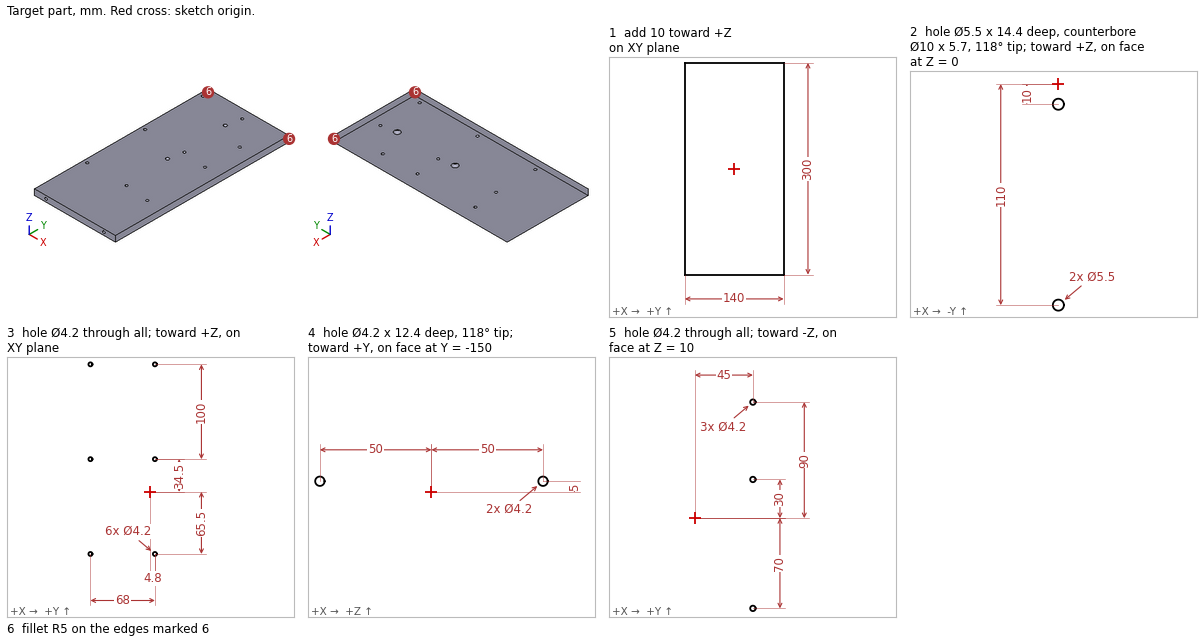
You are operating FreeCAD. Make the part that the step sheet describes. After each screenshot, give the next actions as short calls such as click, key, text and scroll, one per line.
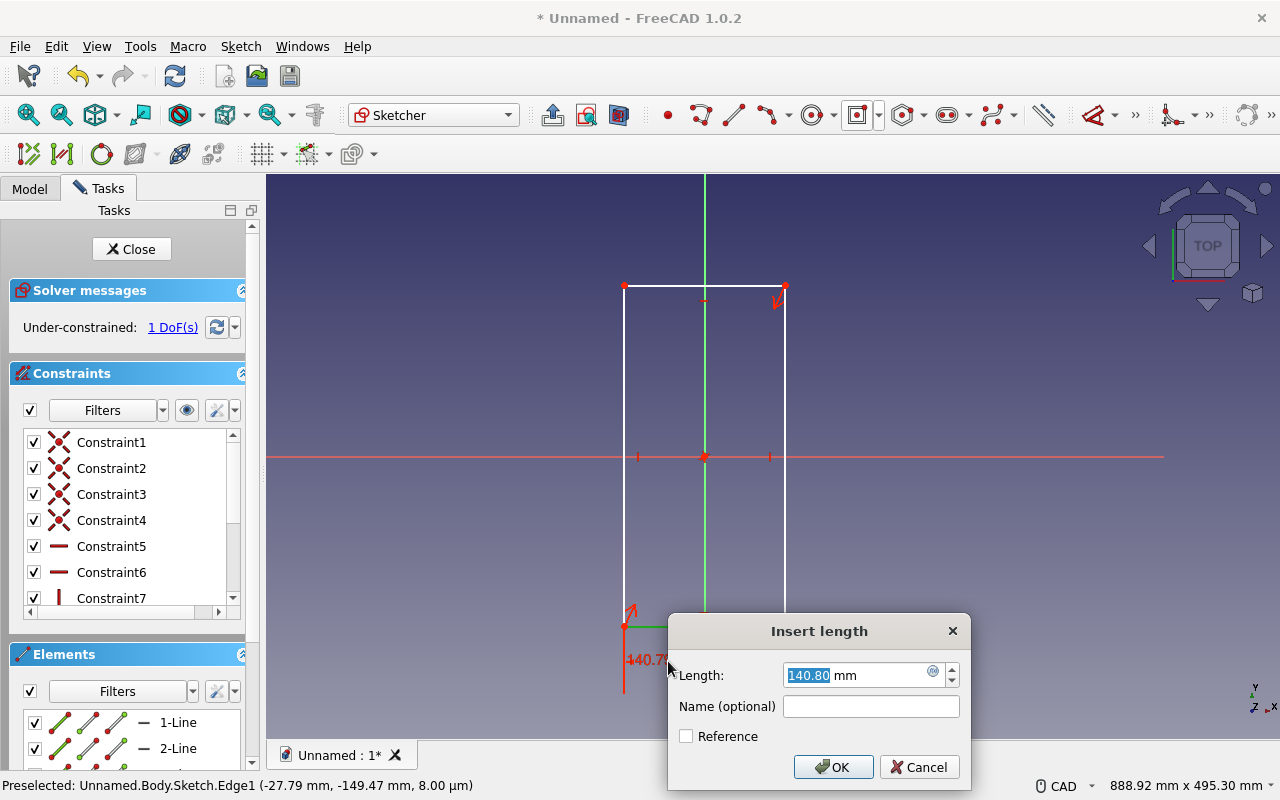
text(140)
key(Return)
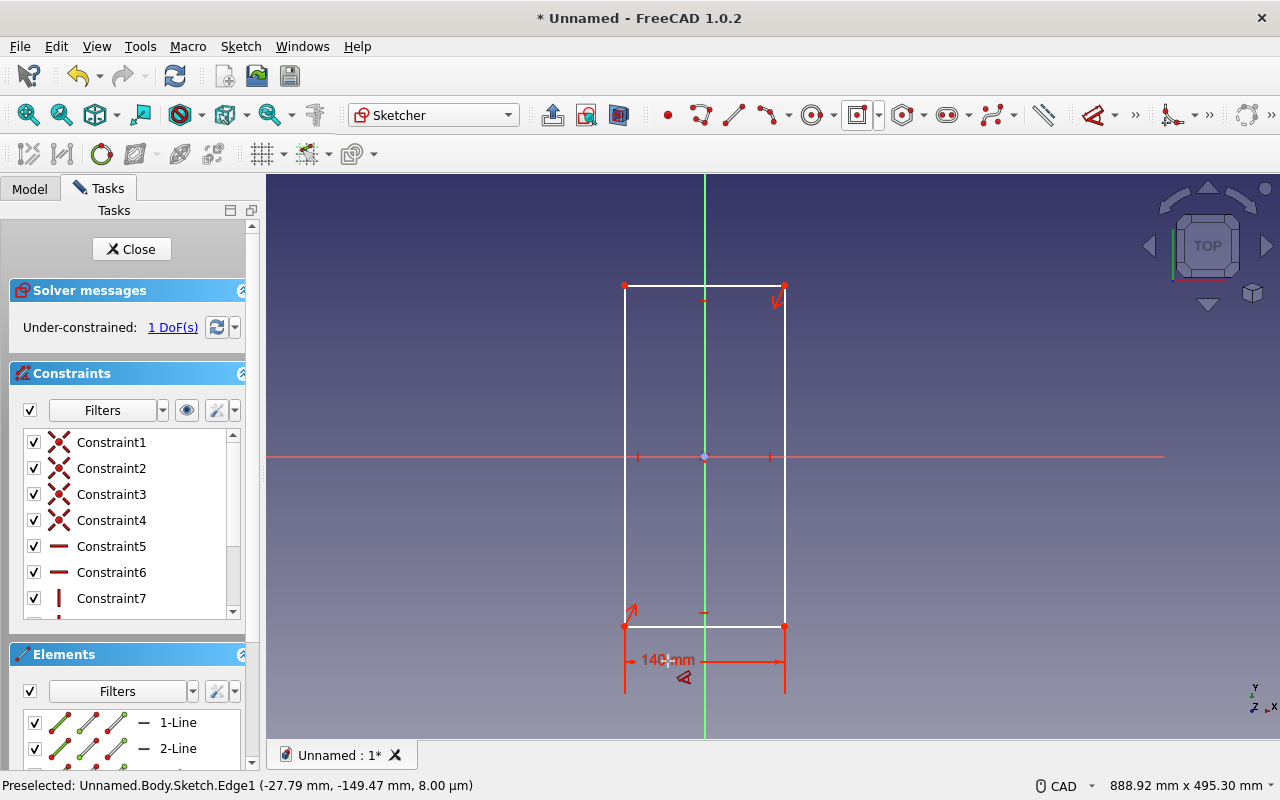
click(785, 525)
click(819, 378)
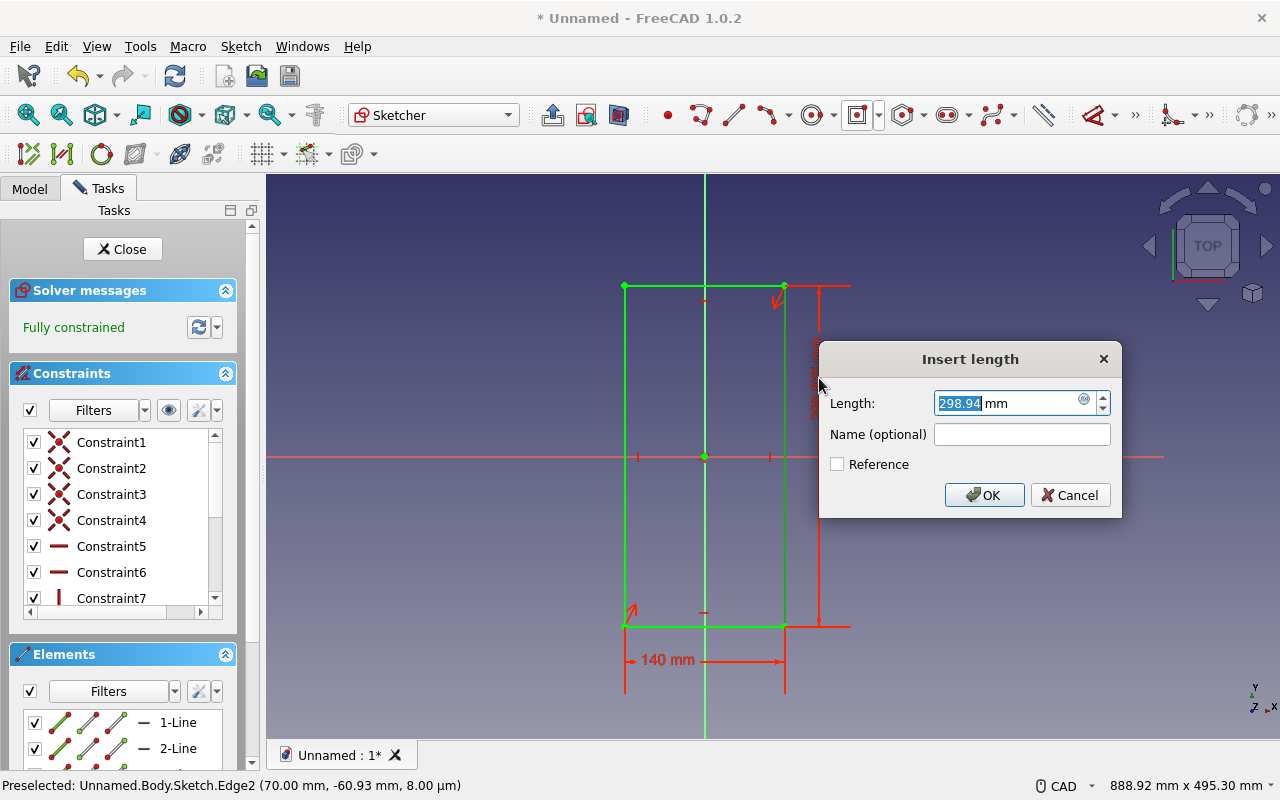
text(300)
key(Return)
key(Escape)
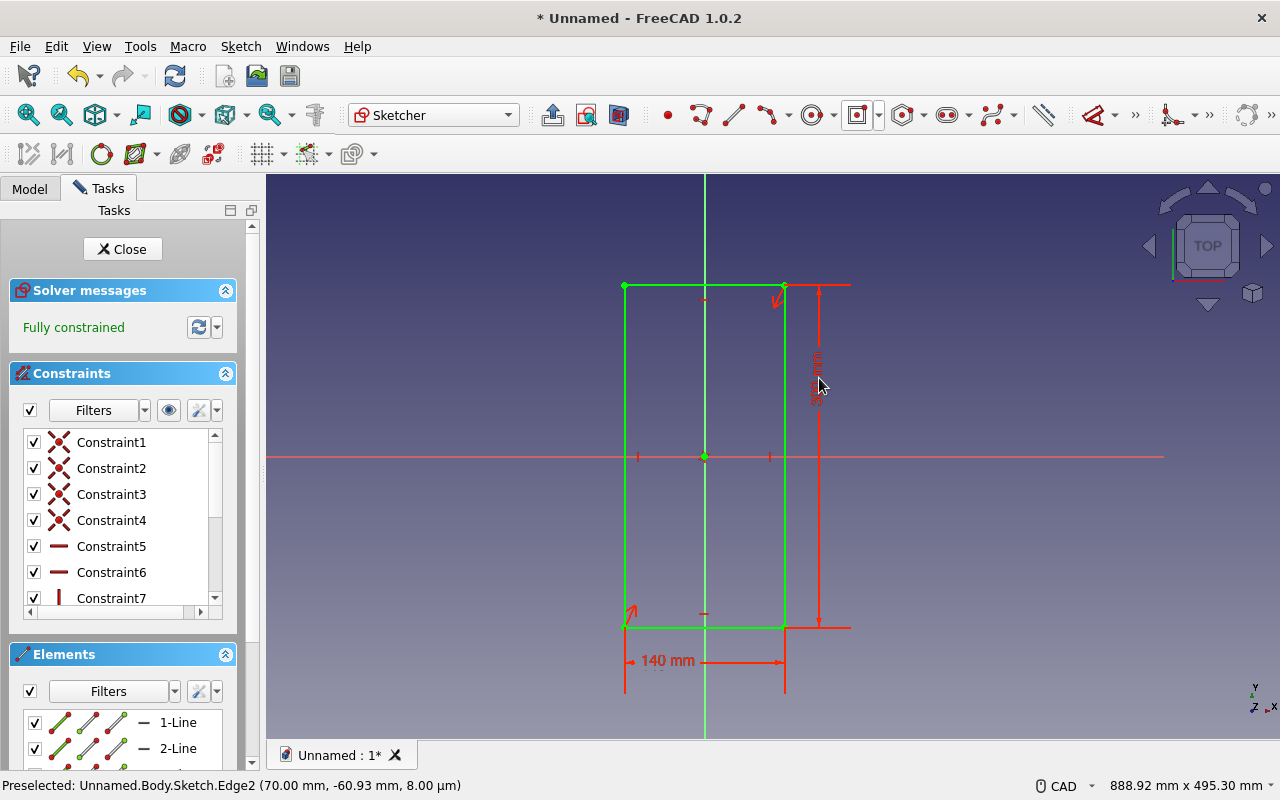
click(123, 249)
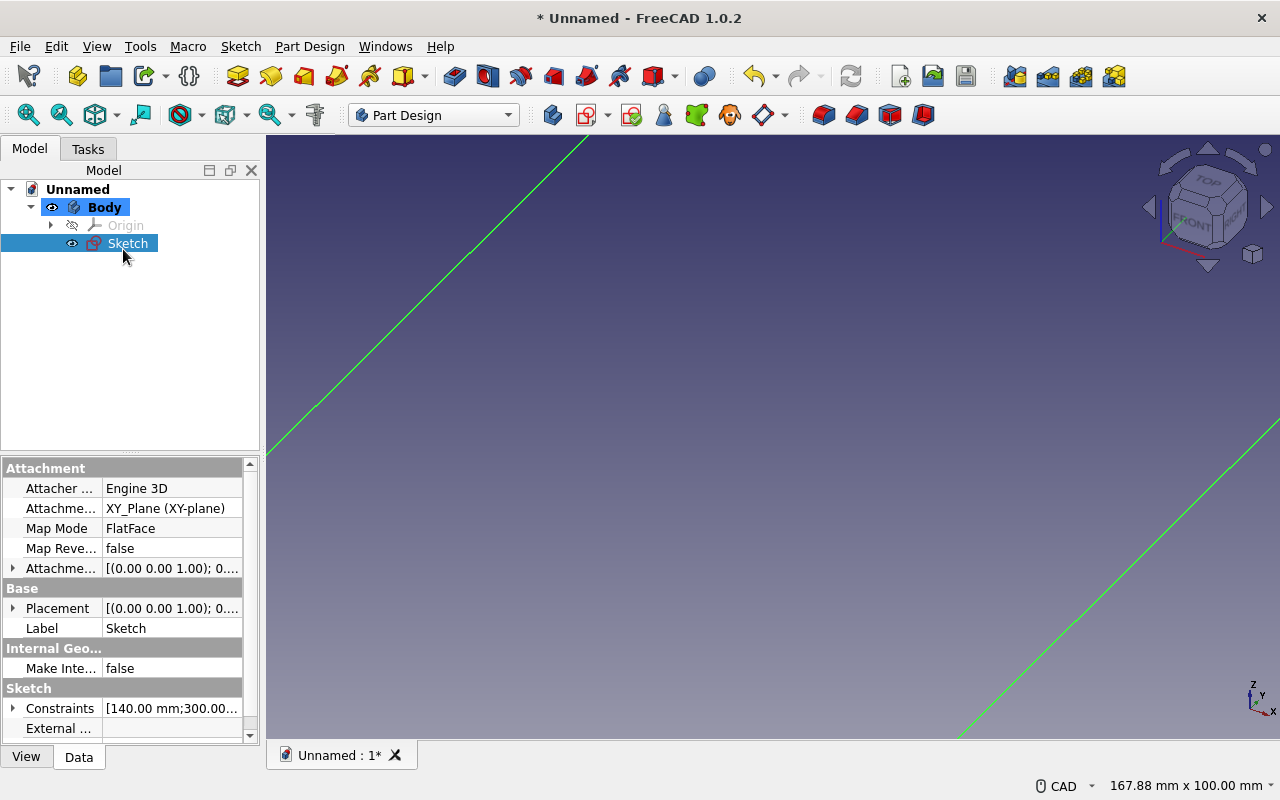
click(238, 76)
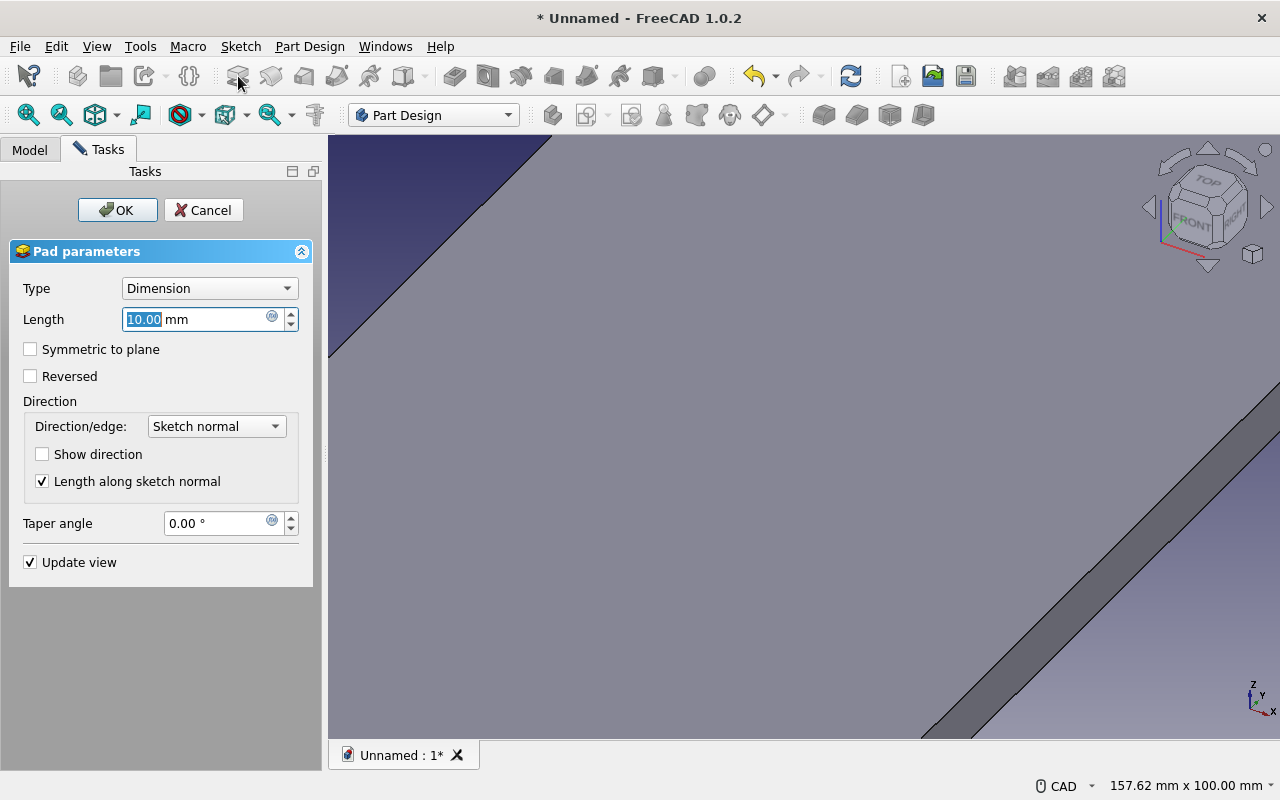
text(10)
key(Tab)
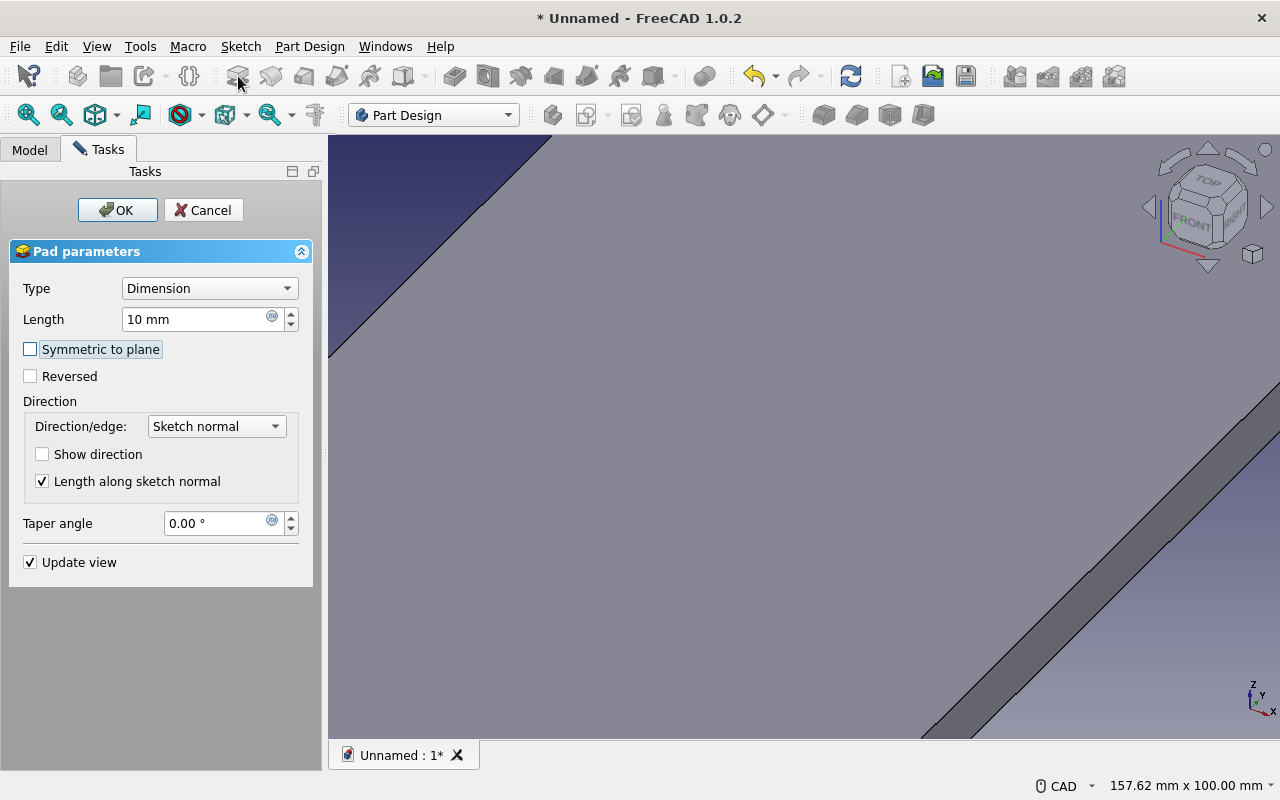
click(118, 210)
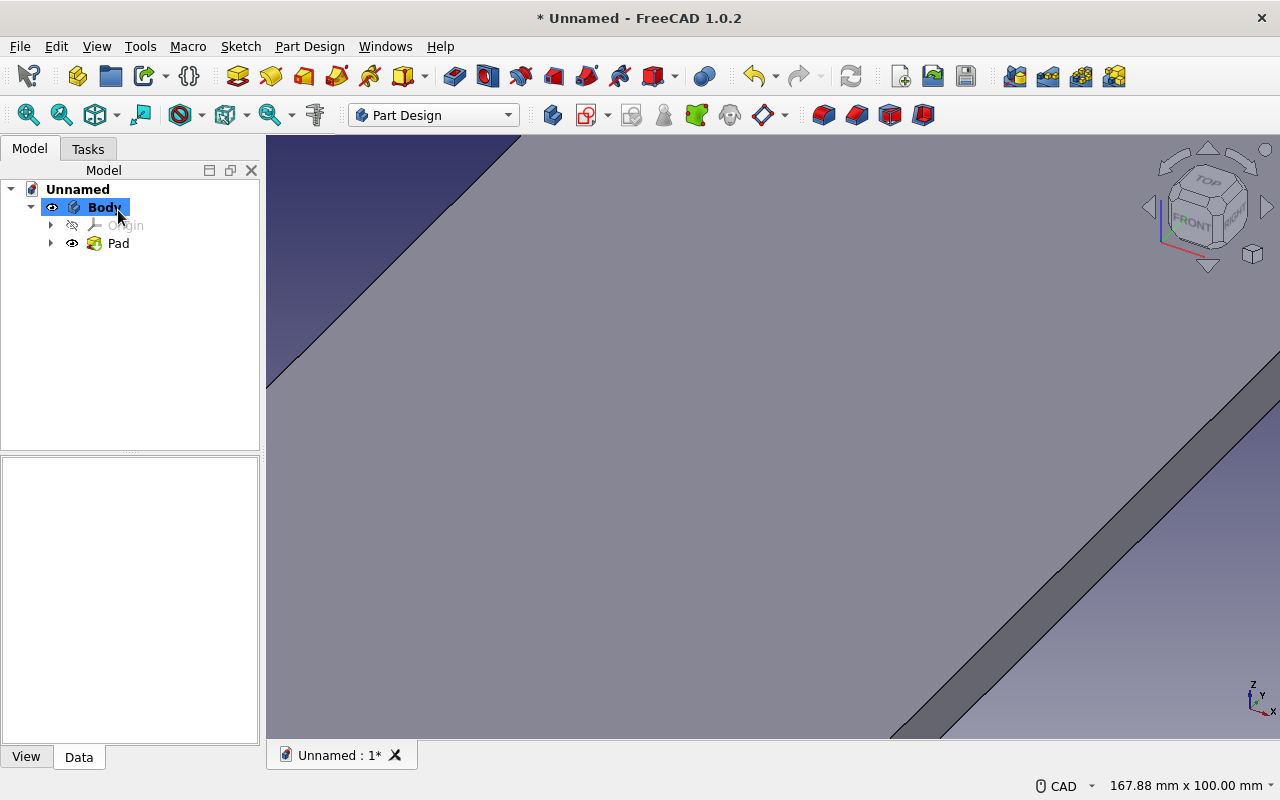
click(29, 116)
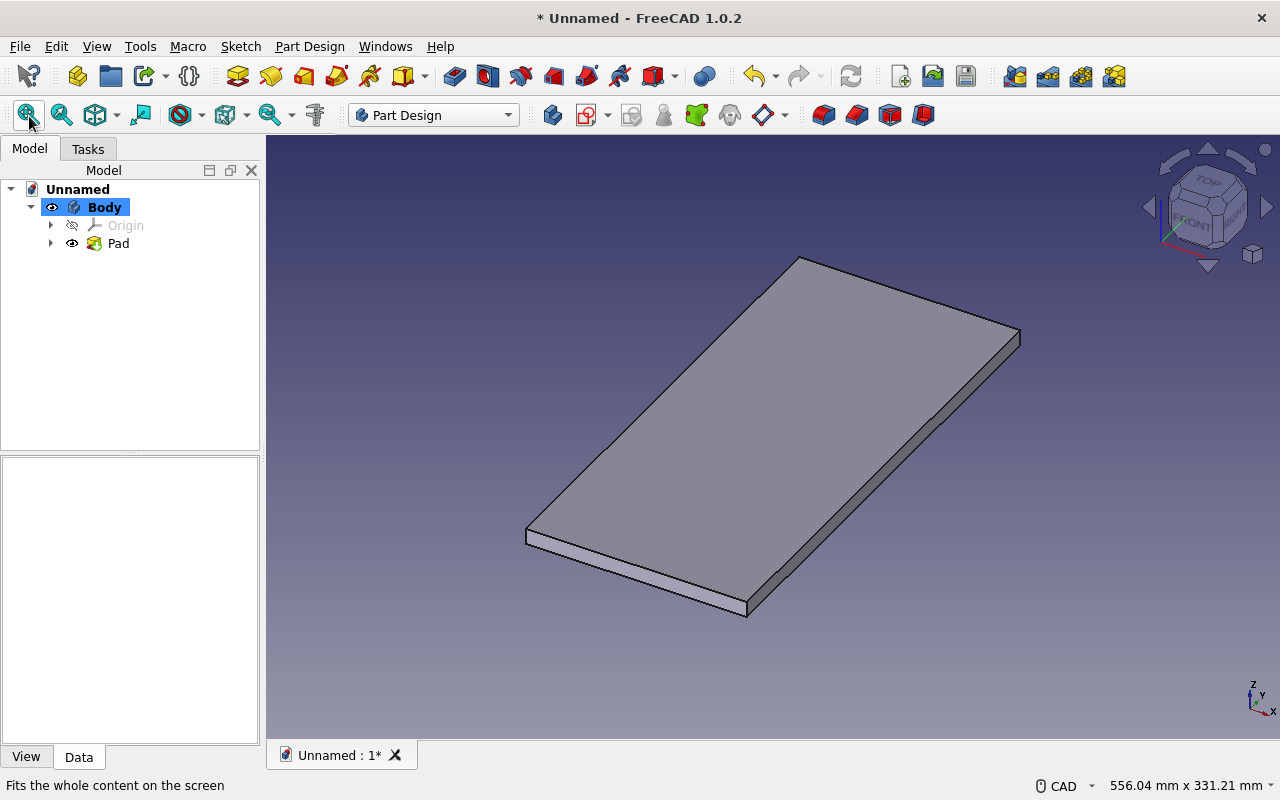
key(5)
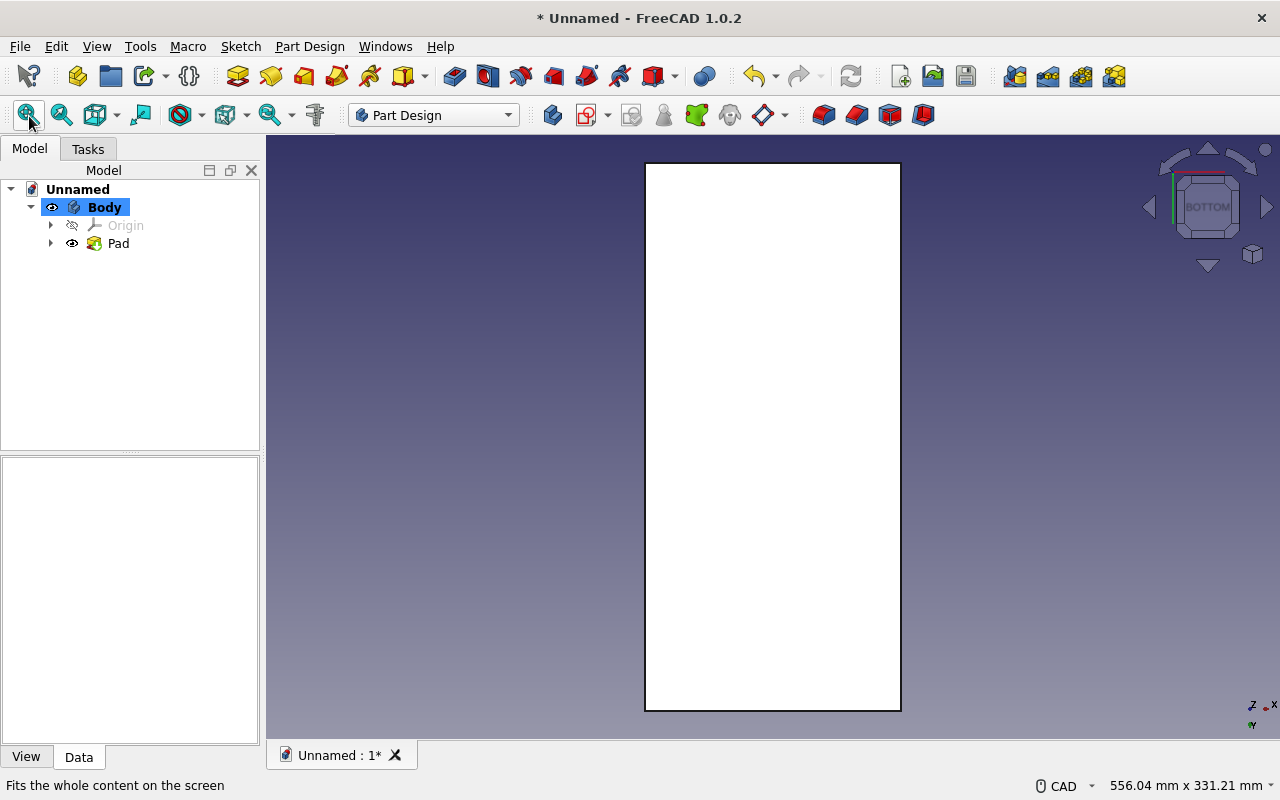
click(773, 514)